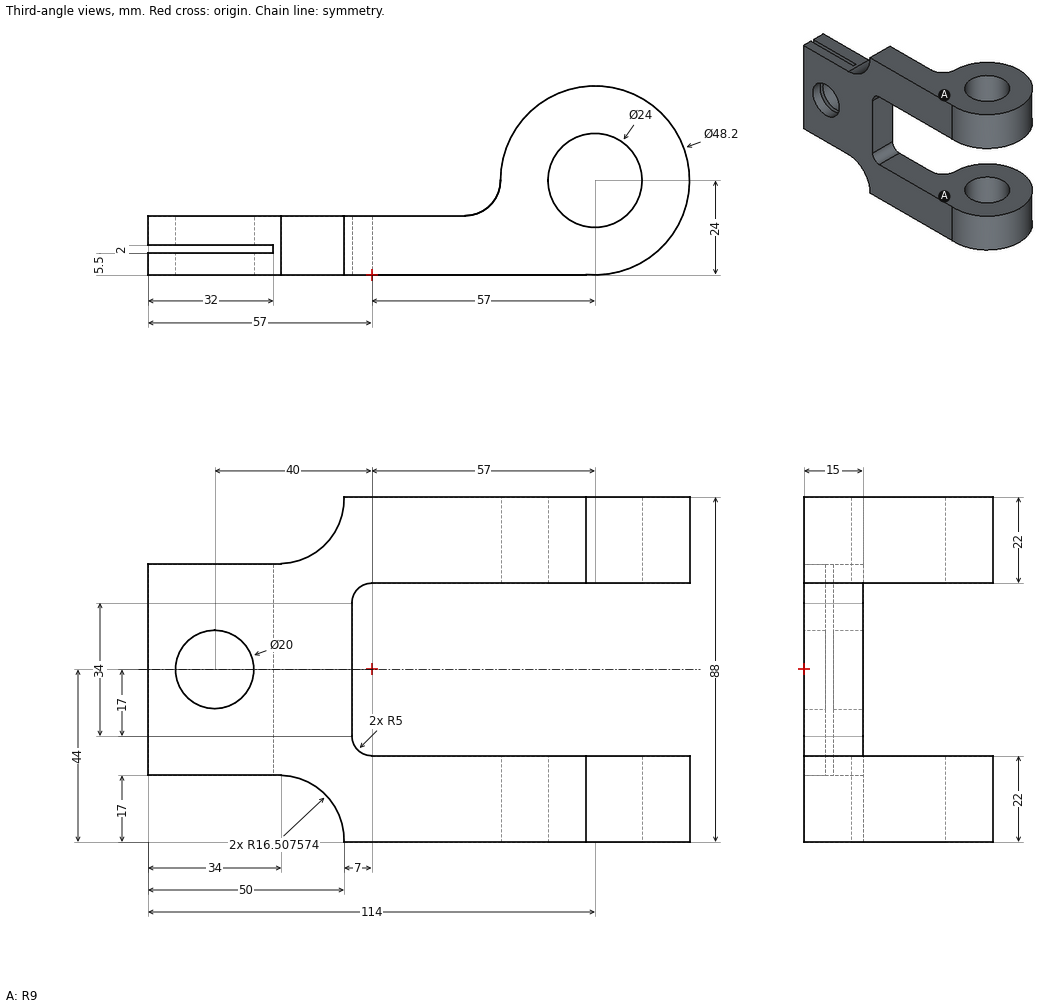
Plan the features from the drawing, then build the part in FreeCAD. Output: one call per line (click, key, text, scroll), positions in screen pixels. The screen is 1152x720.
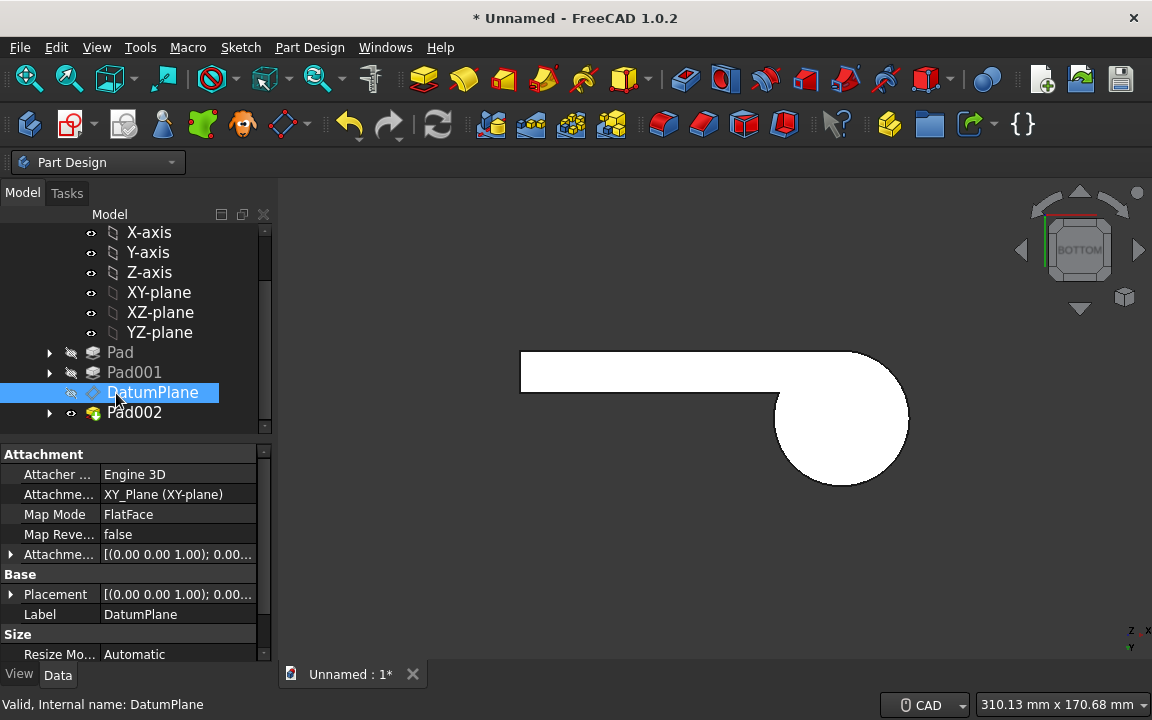
click(826, 417)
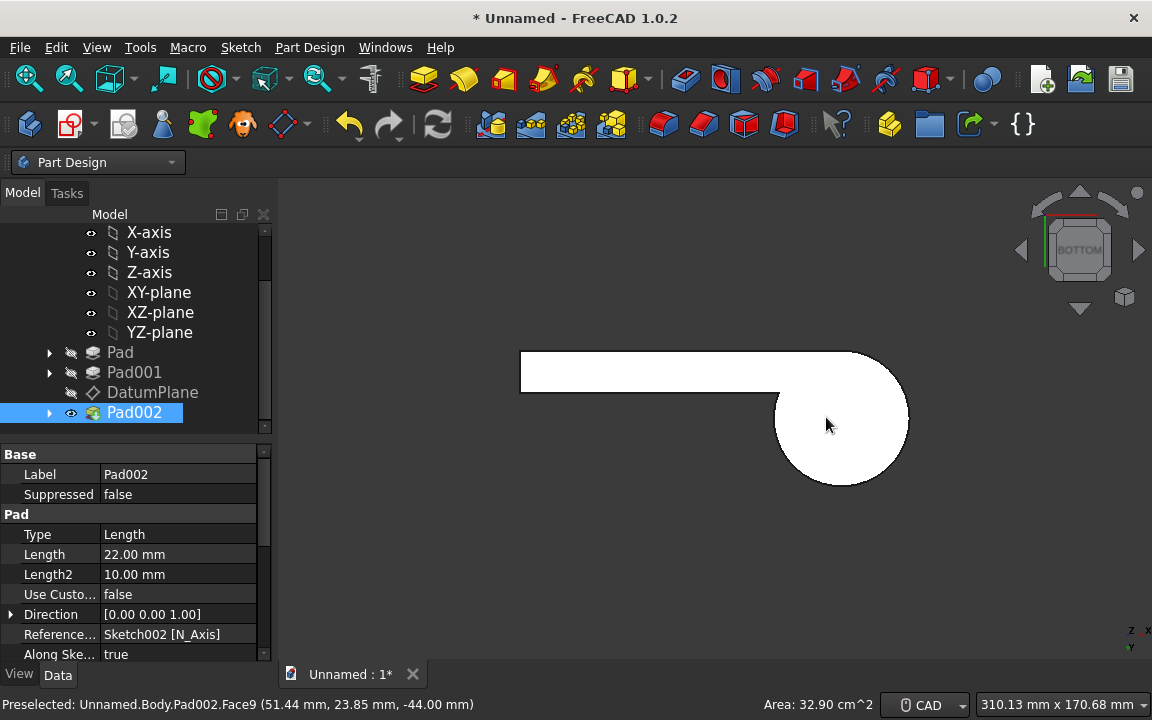
click(70, 124)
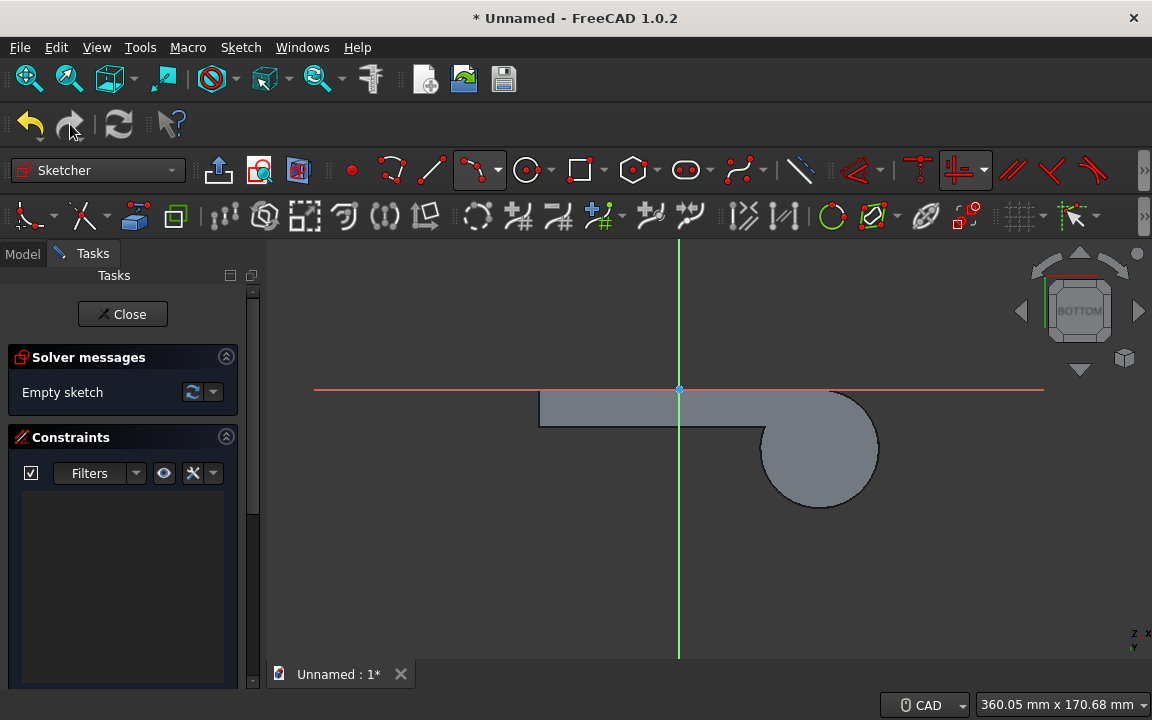
scroll(878, 449, up, 7)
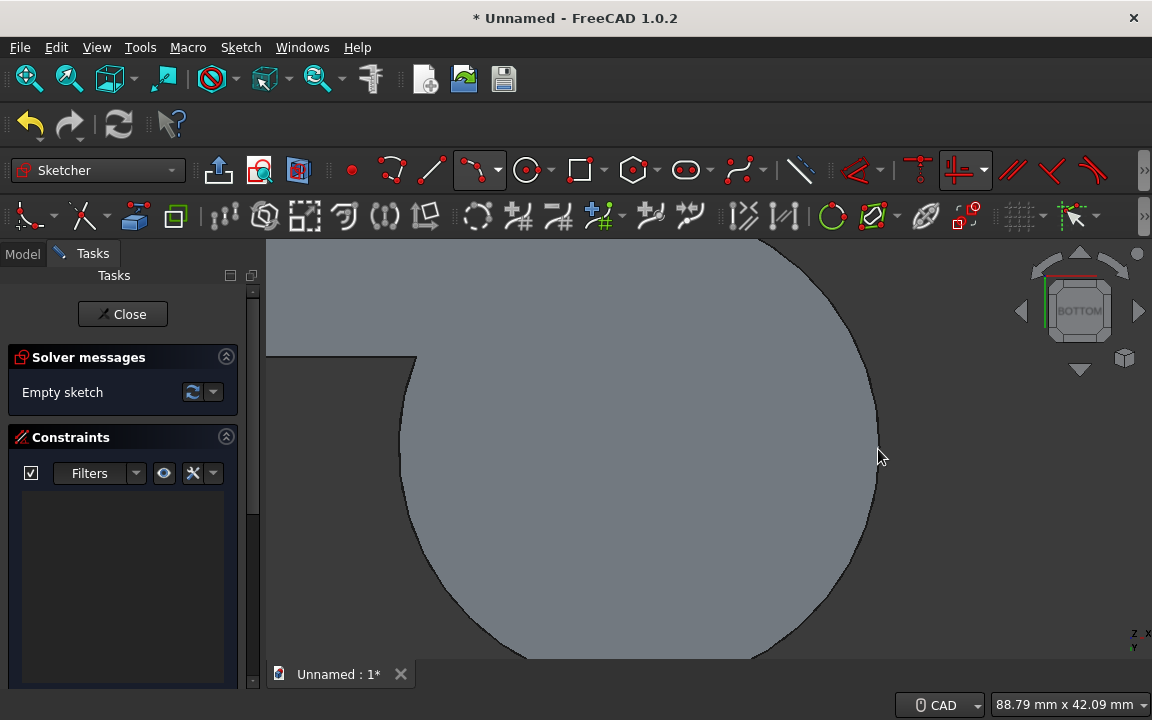
key(g)
key(c)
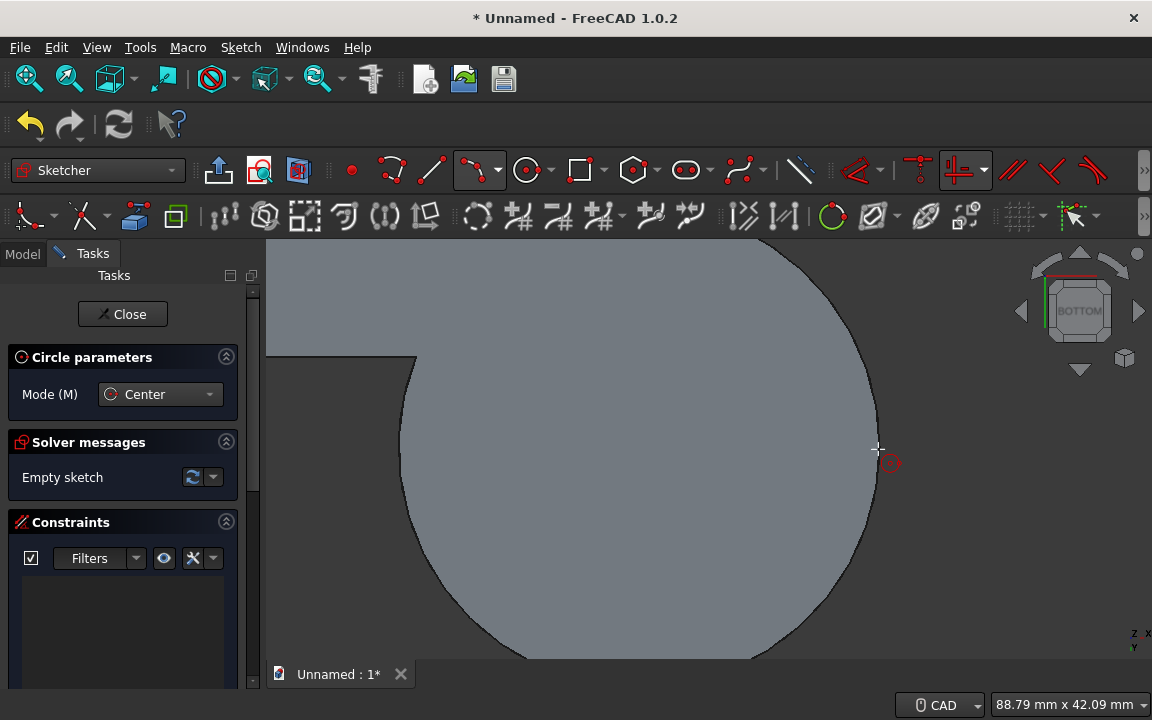
click(639, 447)
move(724, 363)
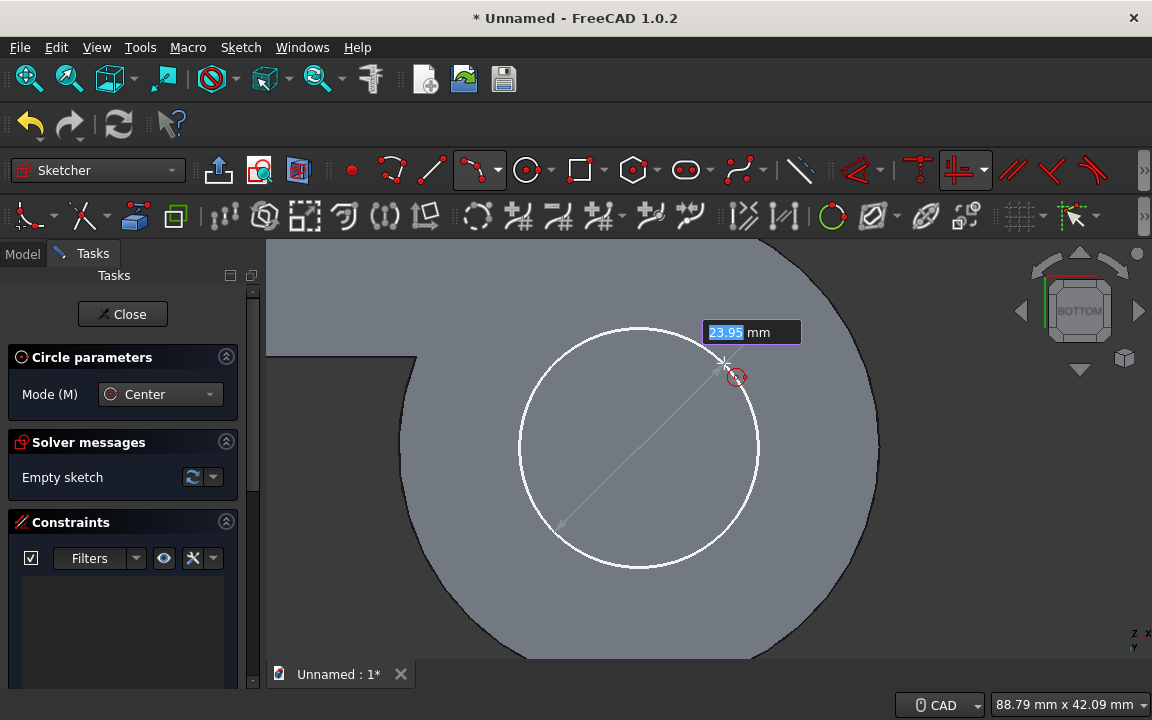
text(24)
key(Return)
key(Escape)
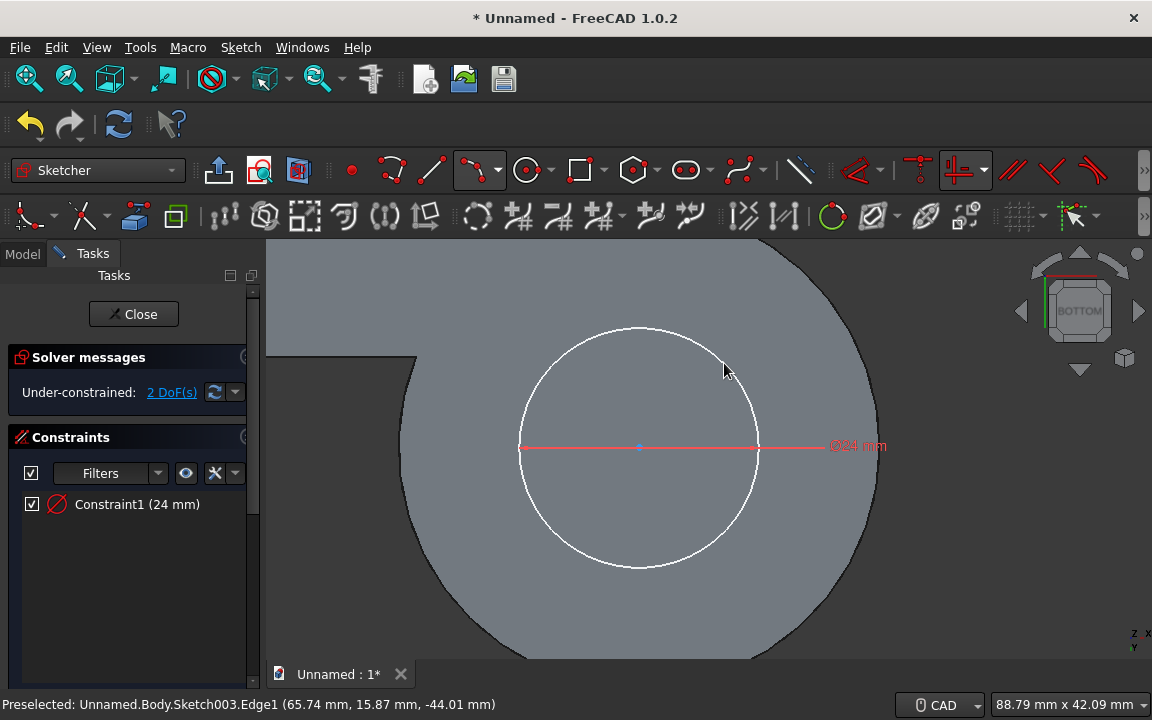
click(856, 170)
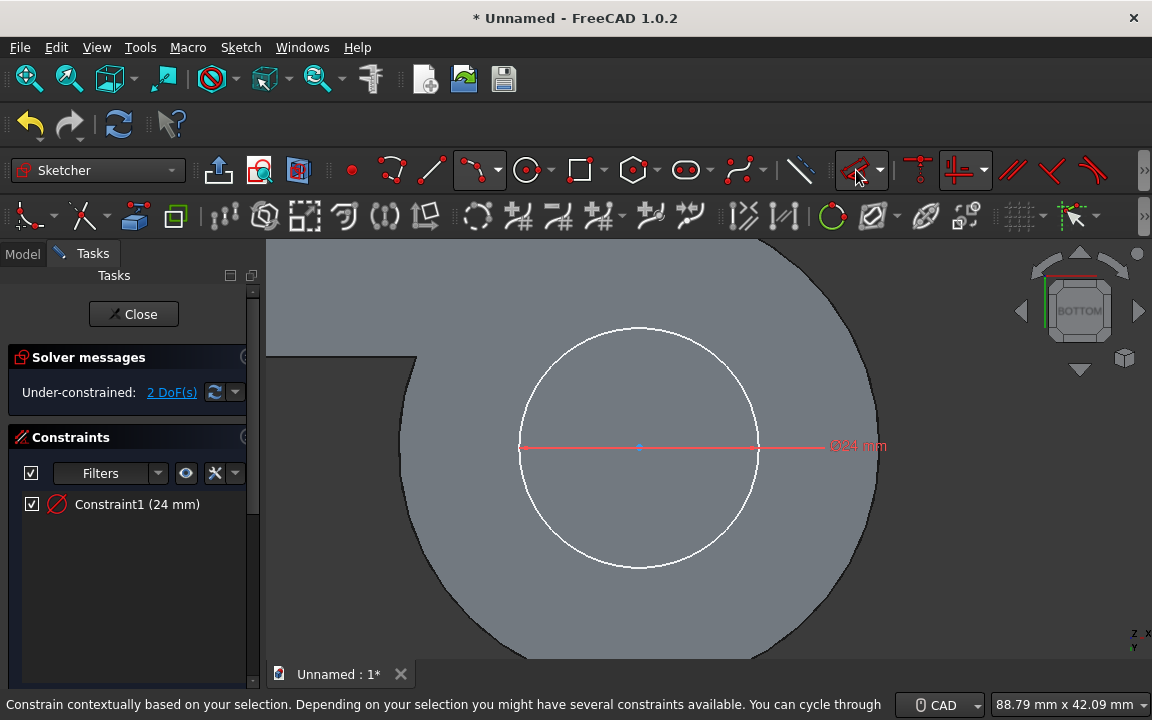
click(639, 448)
click(467, 482)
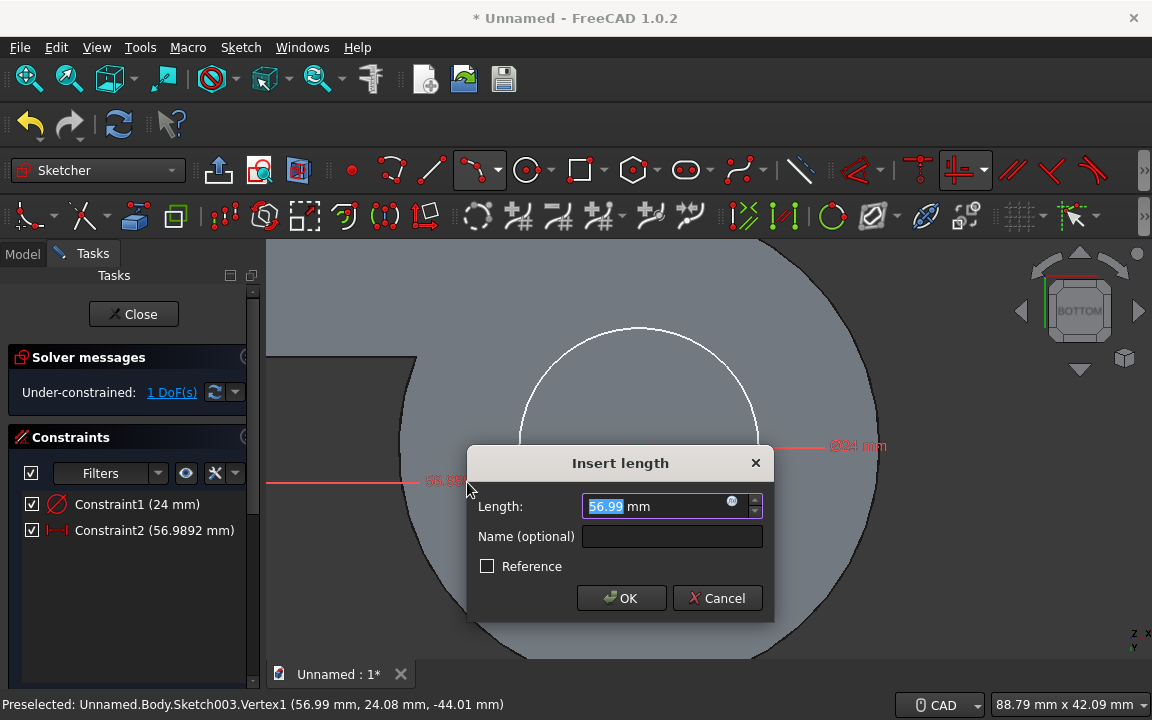
text(57)
key(Return)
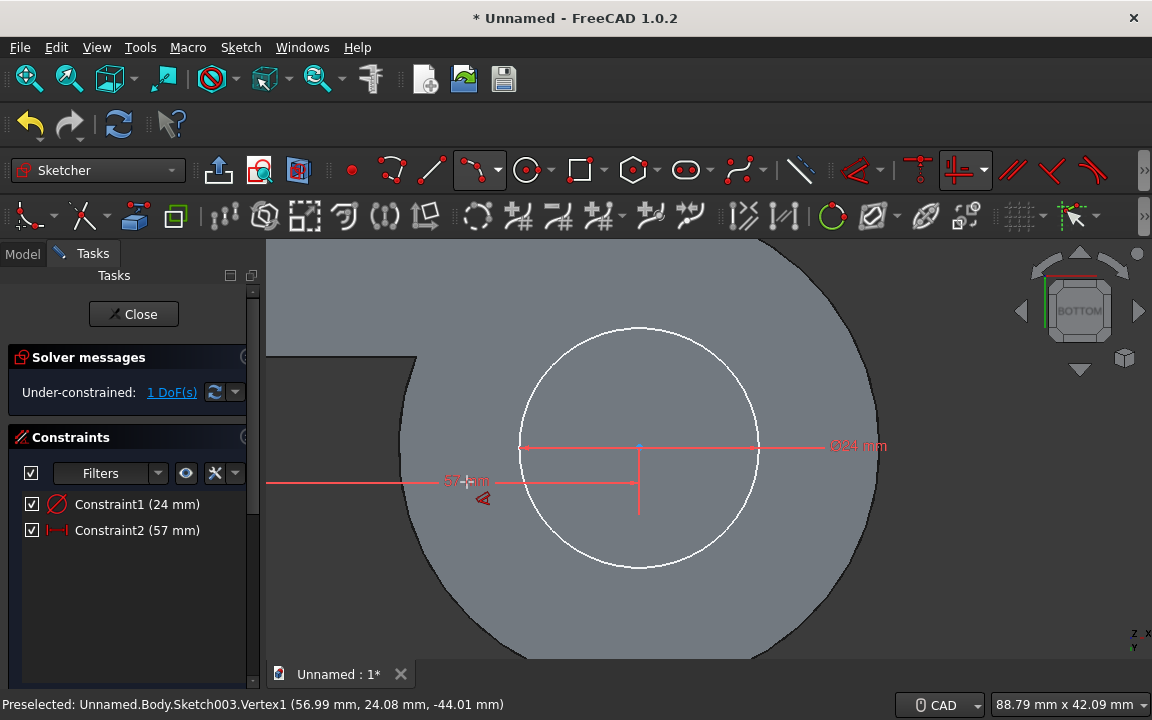
click(639, 448)
click(673, 357)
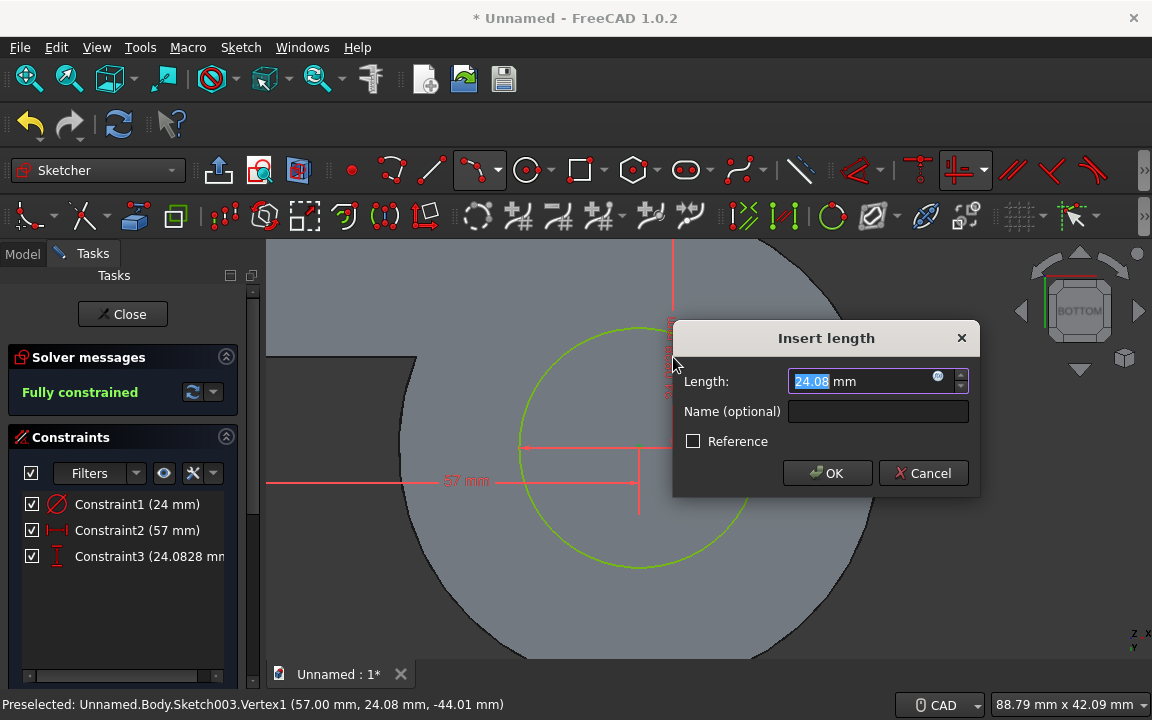
text(24)
key(Return)
key(Escape)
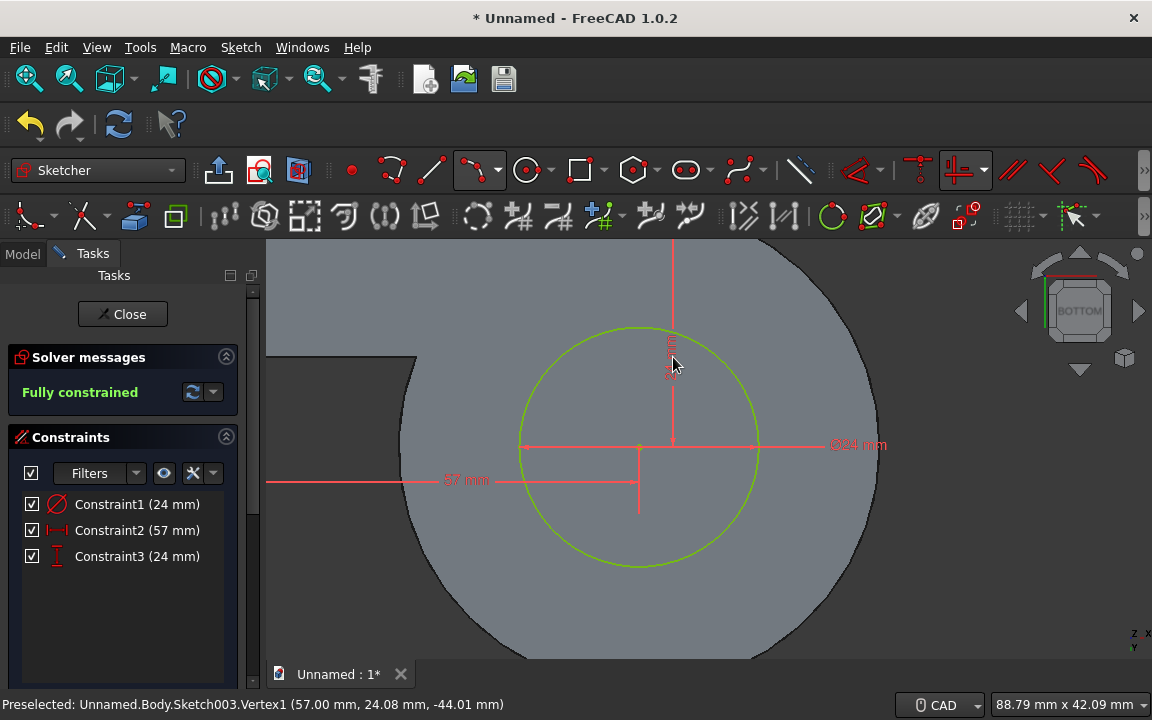
click(123, 314)